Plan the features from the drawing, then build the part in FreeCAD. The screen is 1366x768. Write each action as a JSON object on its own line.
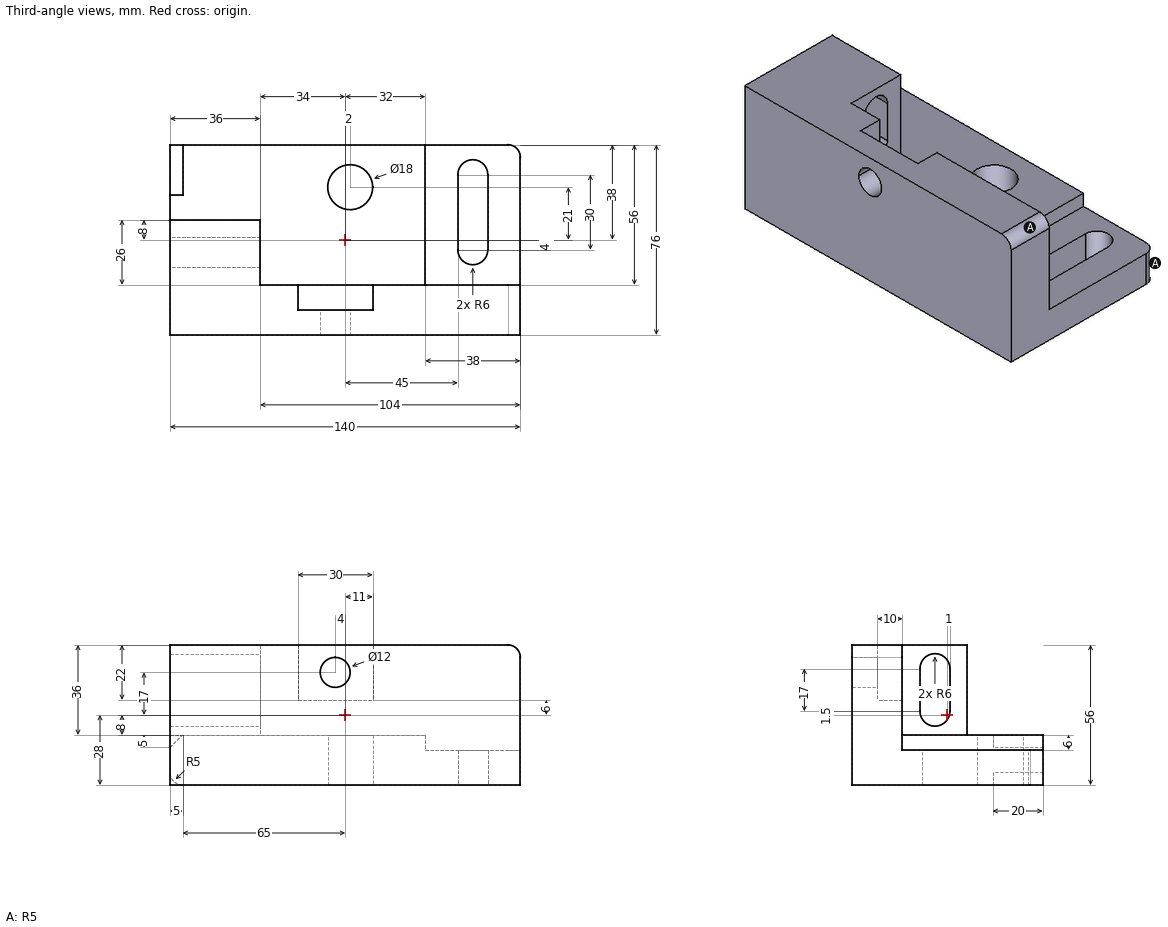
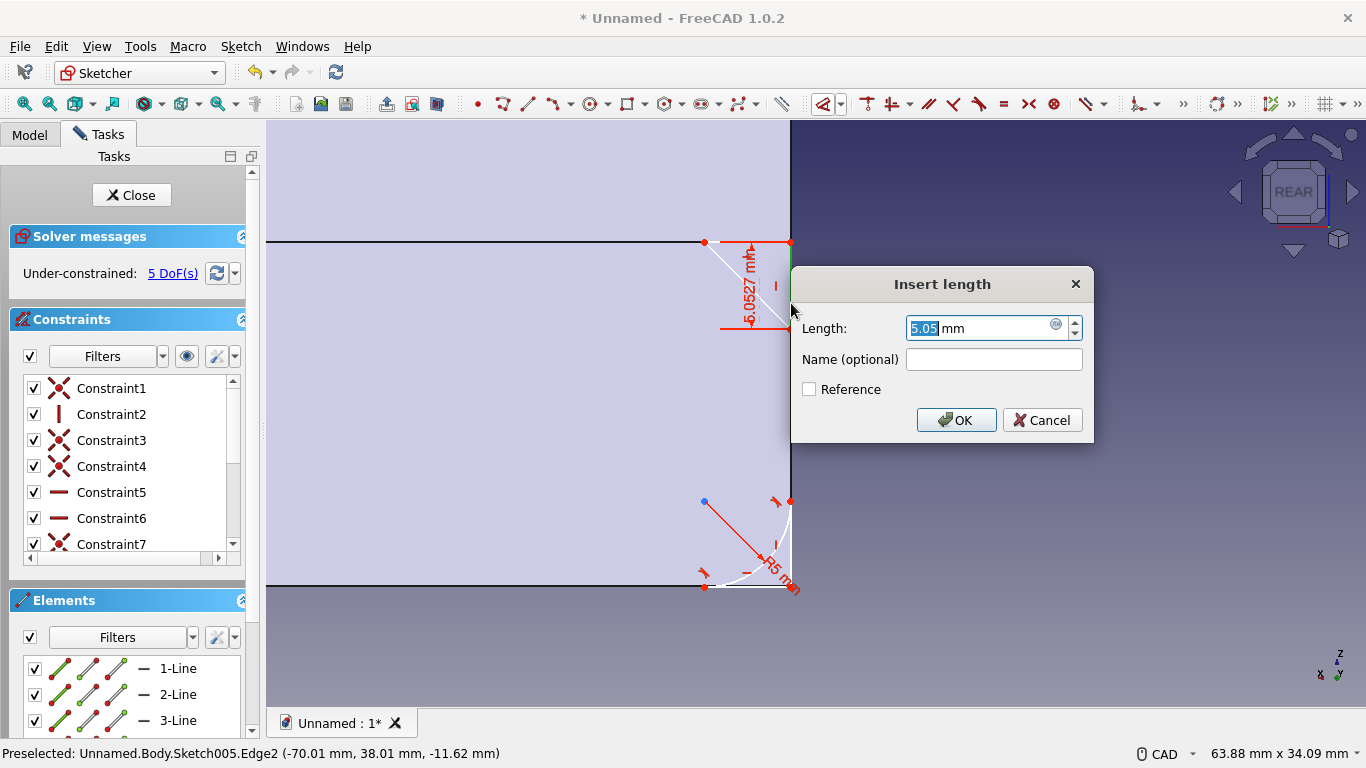
{"action": "type", "text": "5"}
{"action": "key", "text": "Return"}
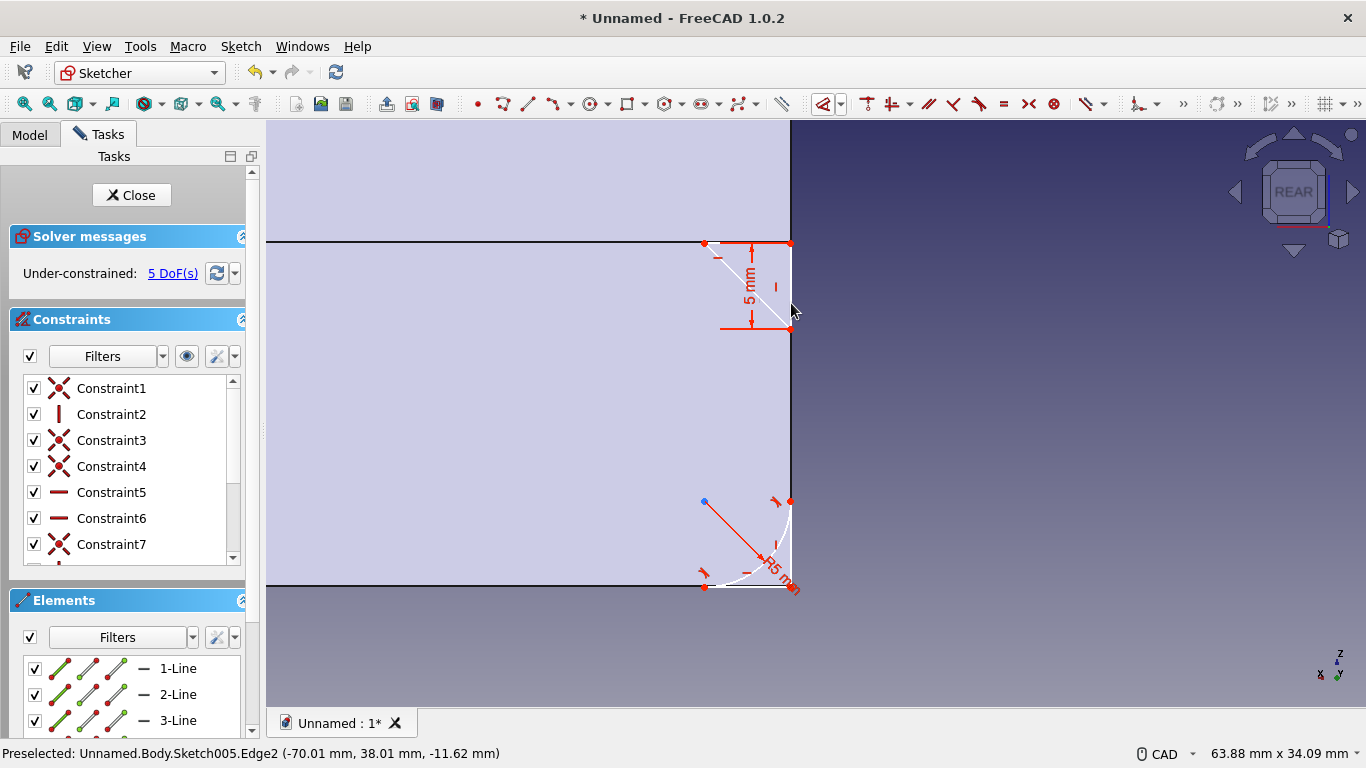
{"action": "left_click", "coordinate": [765, 243]}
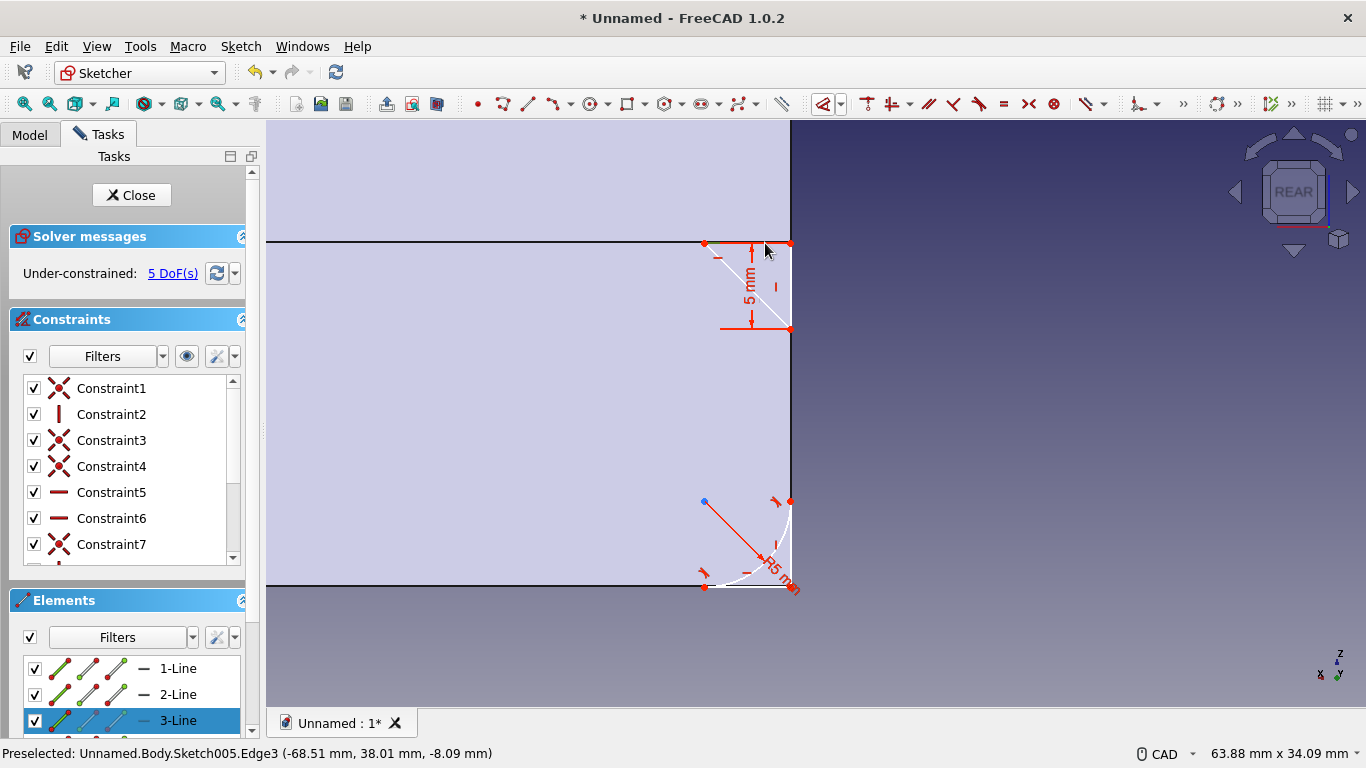
{"action": "key", "text": "l"}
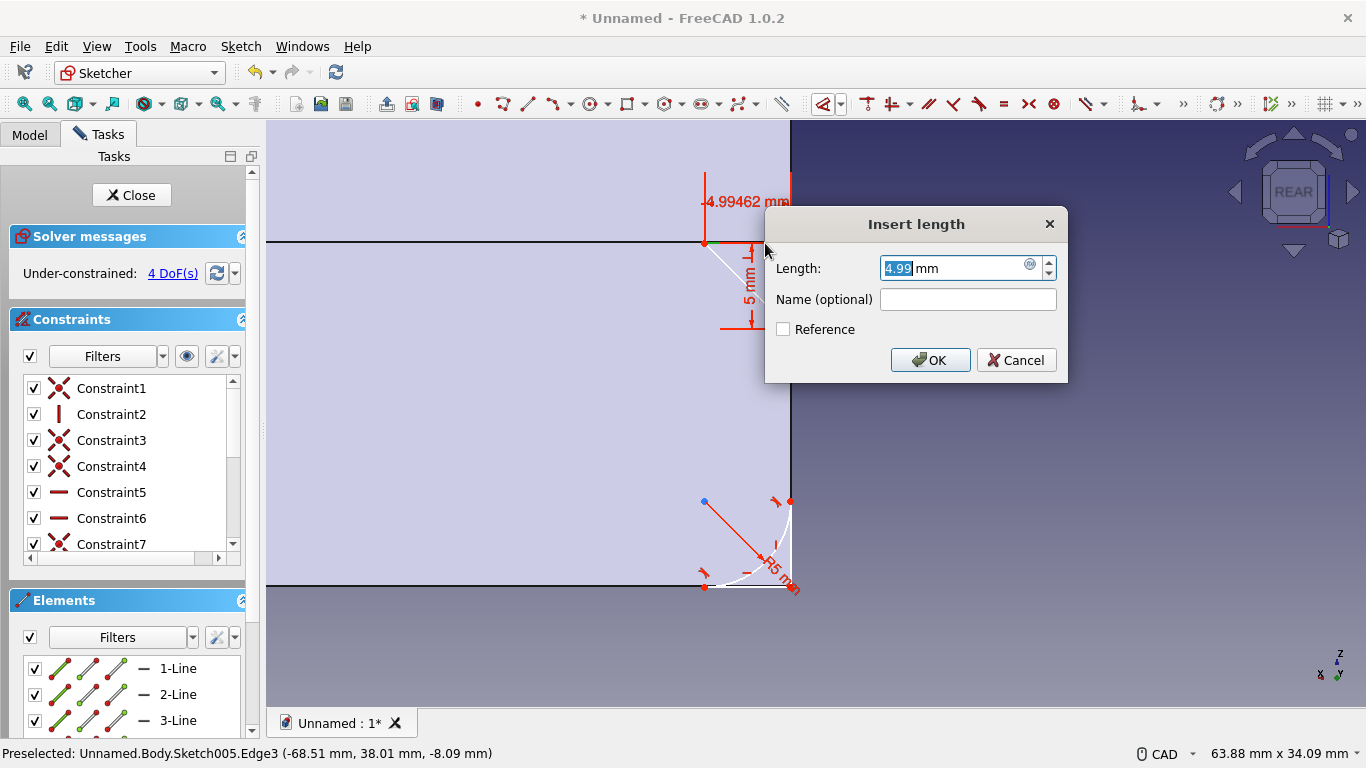
{"action": "type", "text": "5"}
{"action": "key", "text": "Return"}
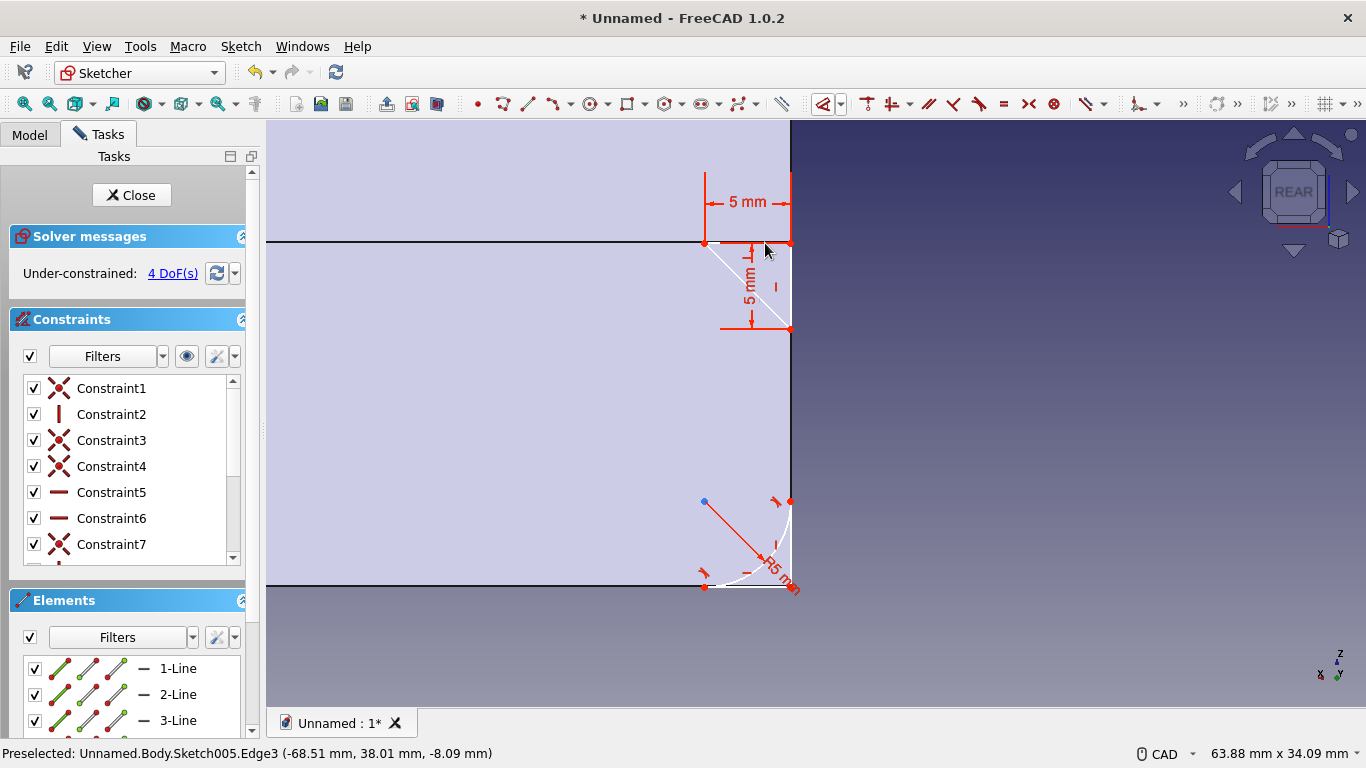
{"action": "left_click", "coordinate": [705, 243]}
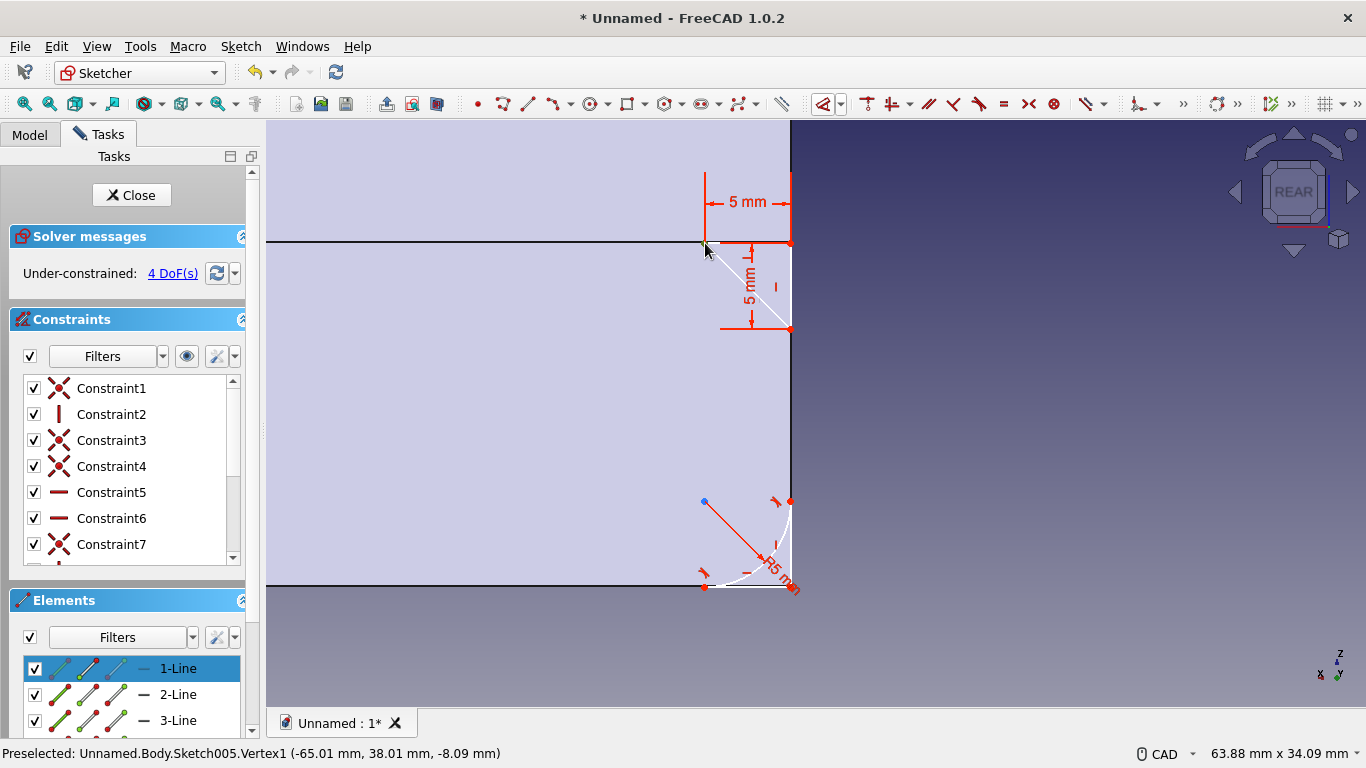
{"action": "key", "text": "i"}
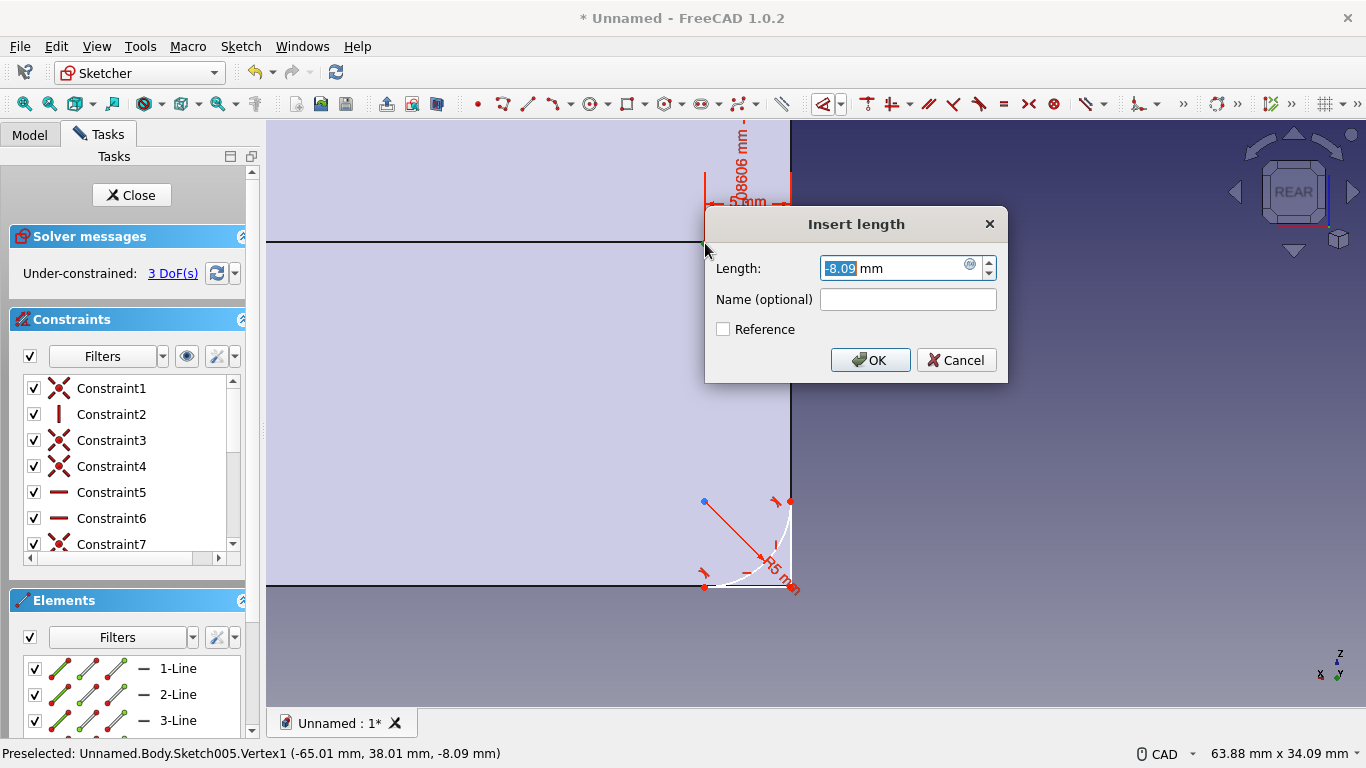
{"action": "type", "text": "-8"}
{"action": "key", "text": "Return"}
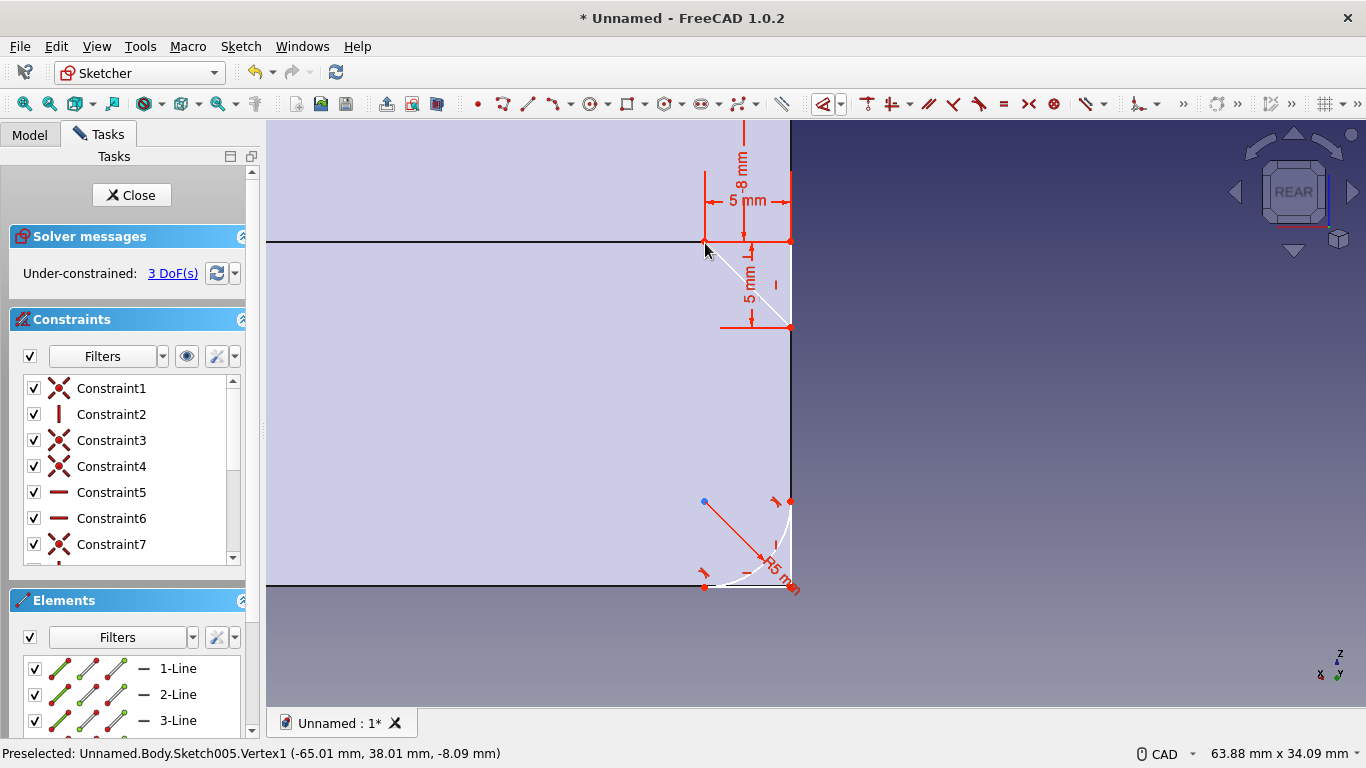
{"action": "left_click", "coordinate": [705, 242]}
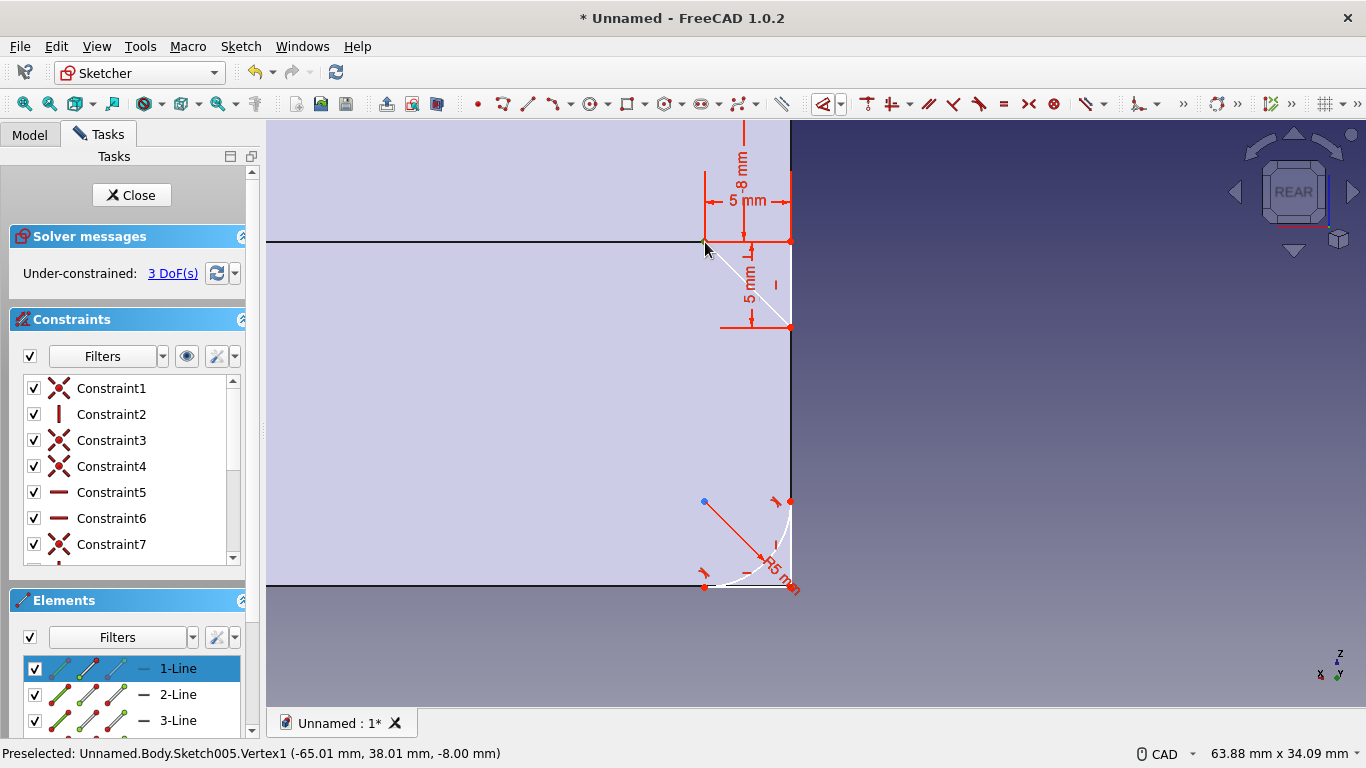
{"action": "left_click", "coordinate": [840, 104]}